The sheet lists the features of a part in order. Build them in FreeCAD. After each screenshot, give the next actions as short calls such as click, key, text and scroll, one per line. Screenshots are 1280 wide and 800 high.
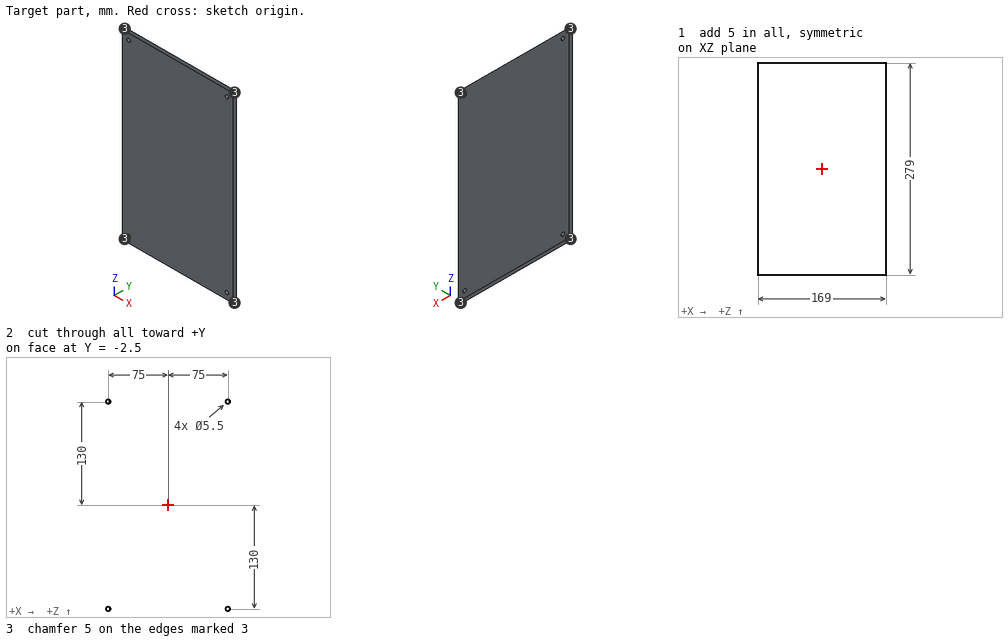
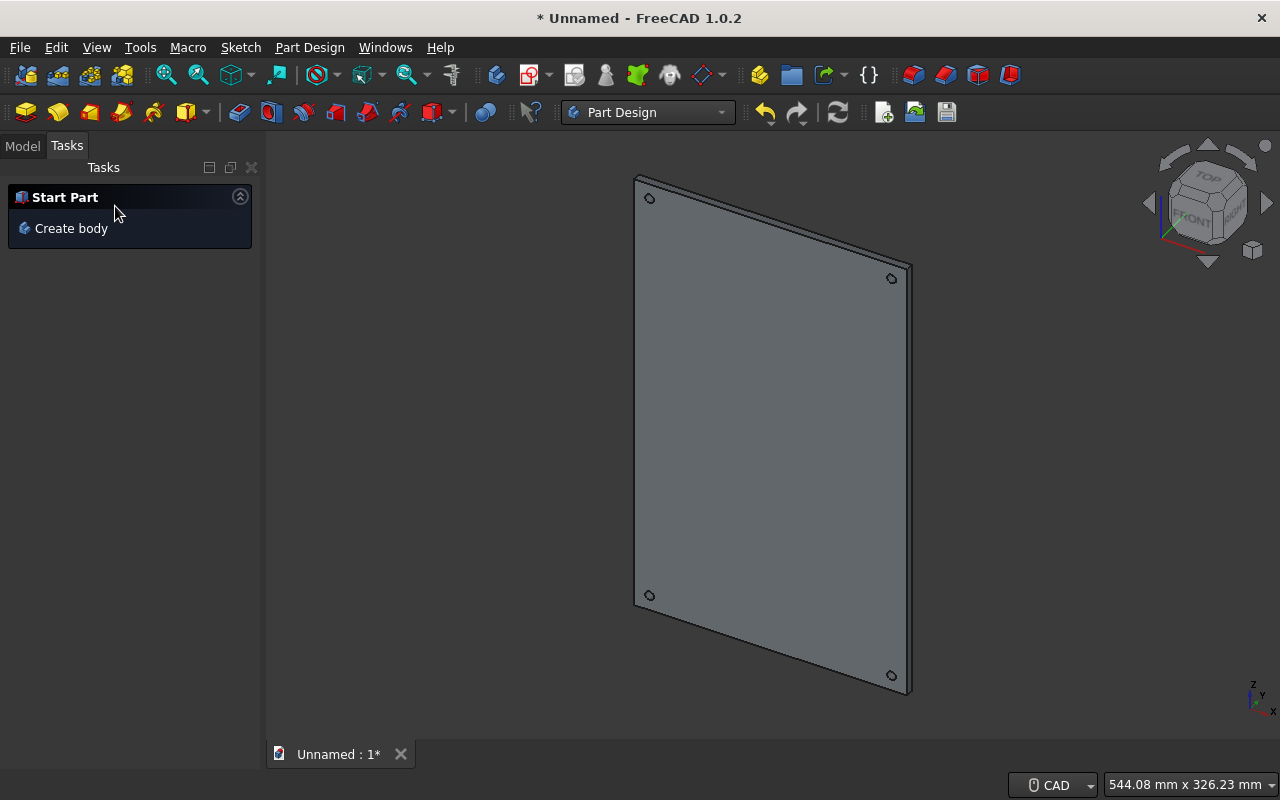
scroll(637, 602, up, 8)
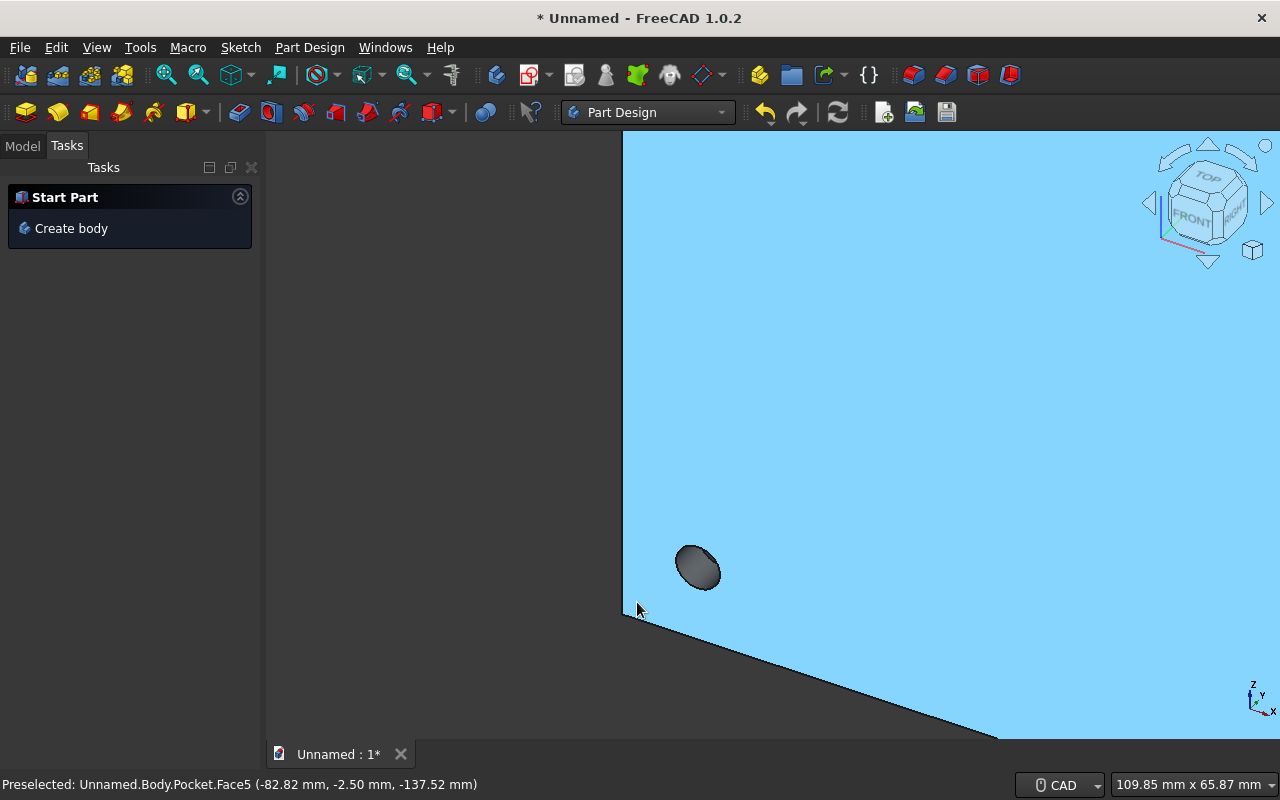
click(168, 76)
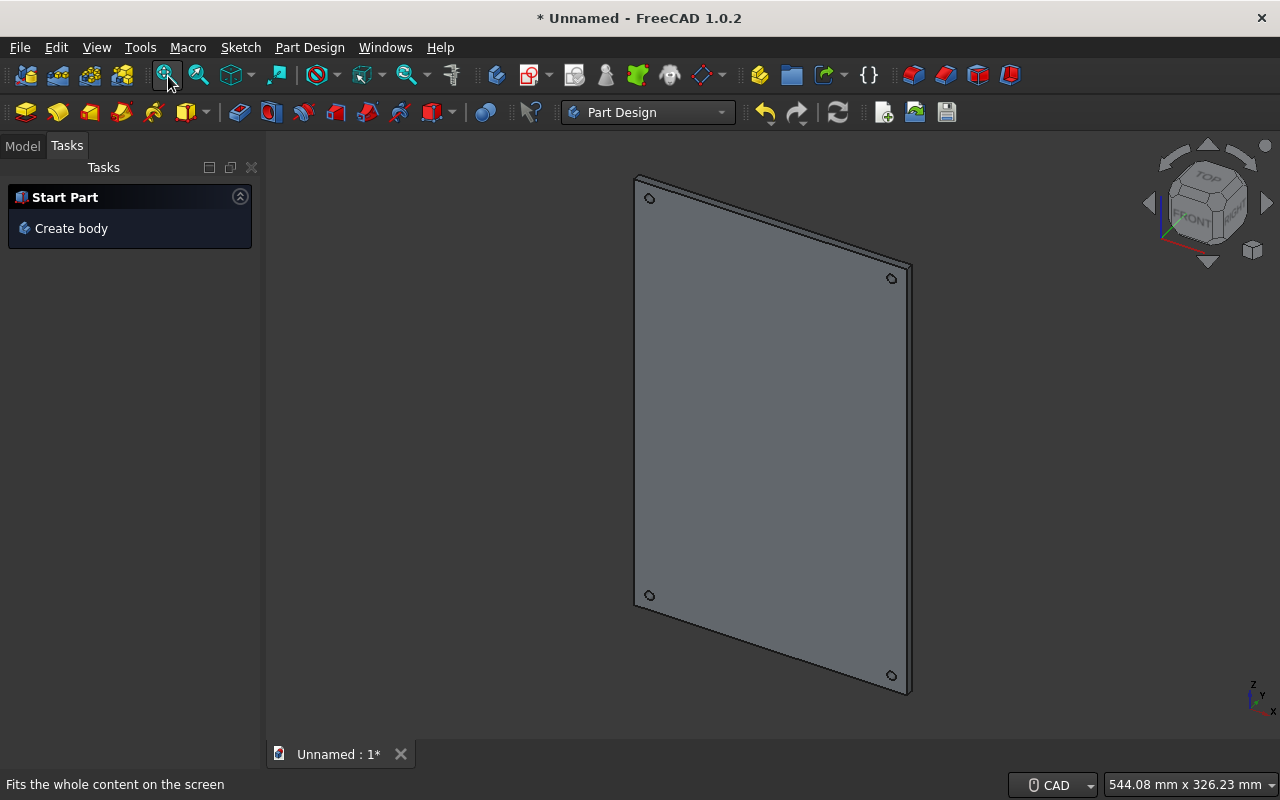
key(0)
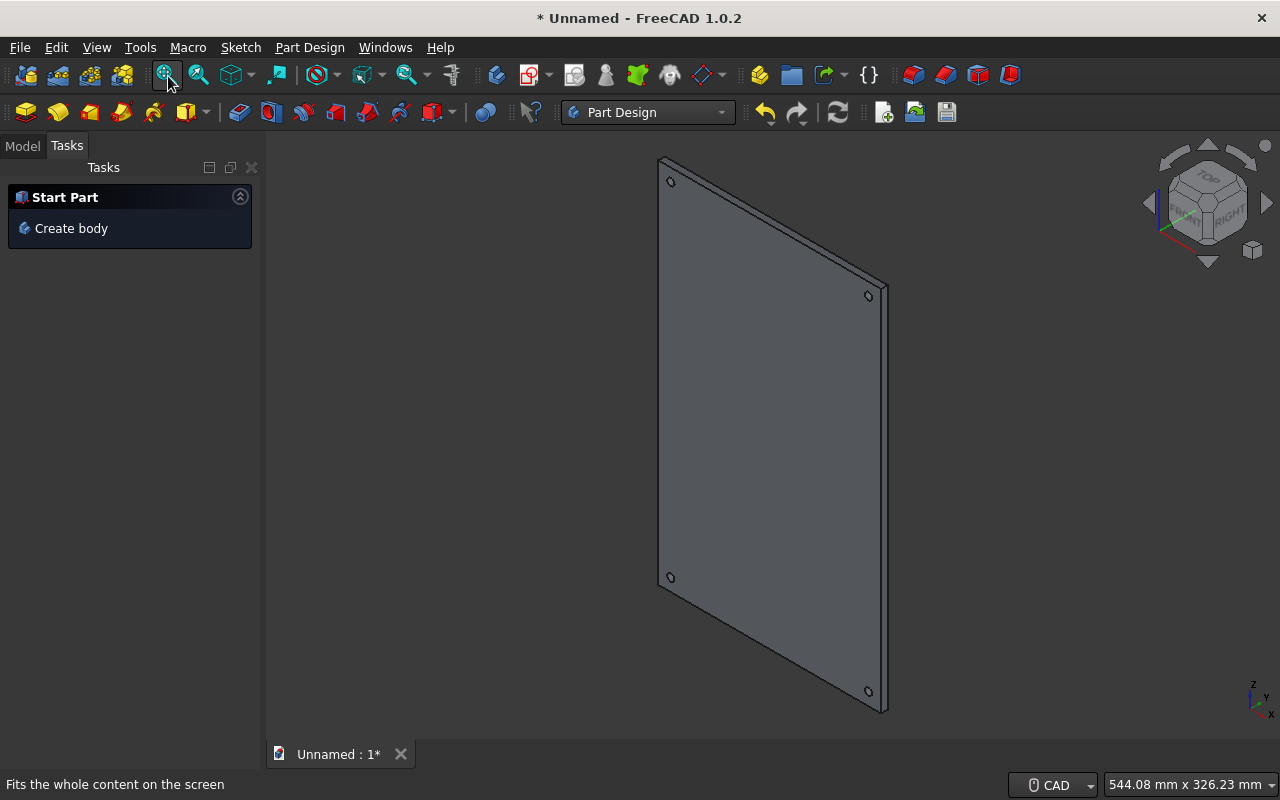
scroll(662, 582, up, 8)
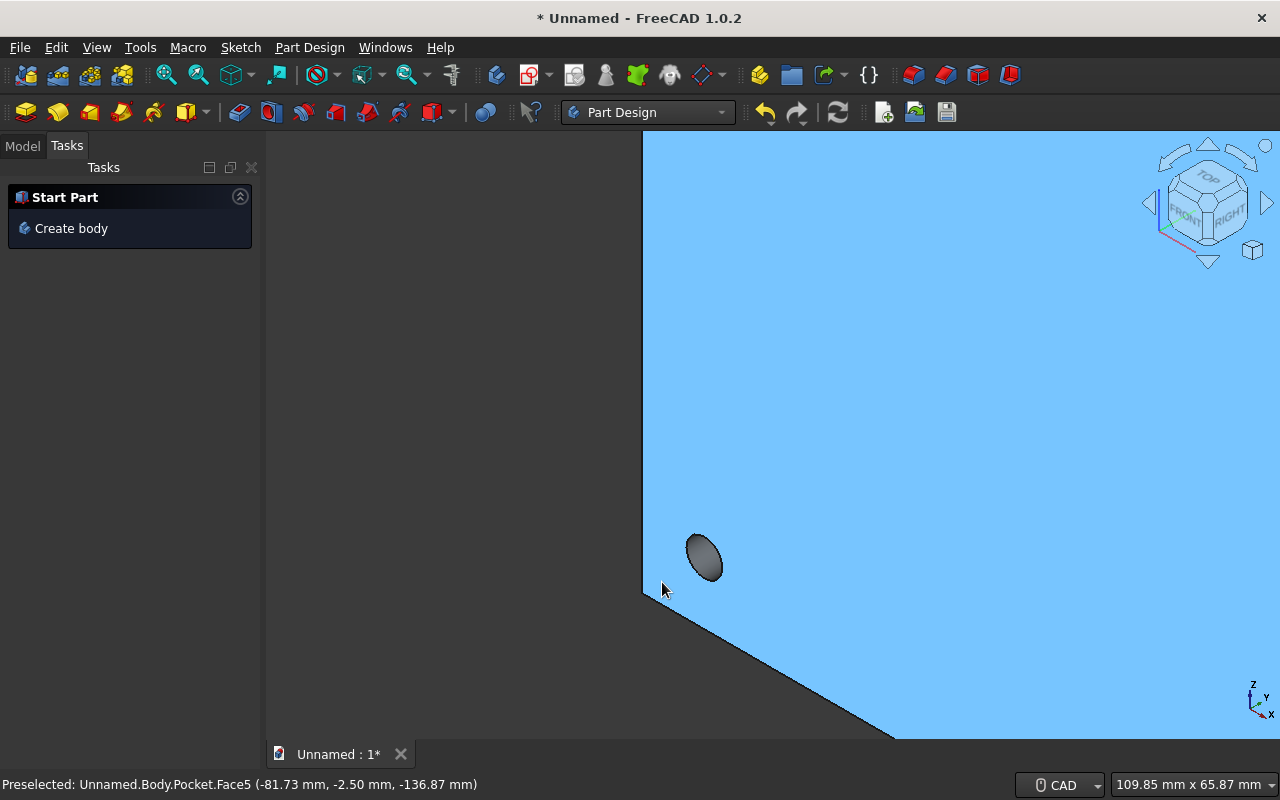
click(168, 76)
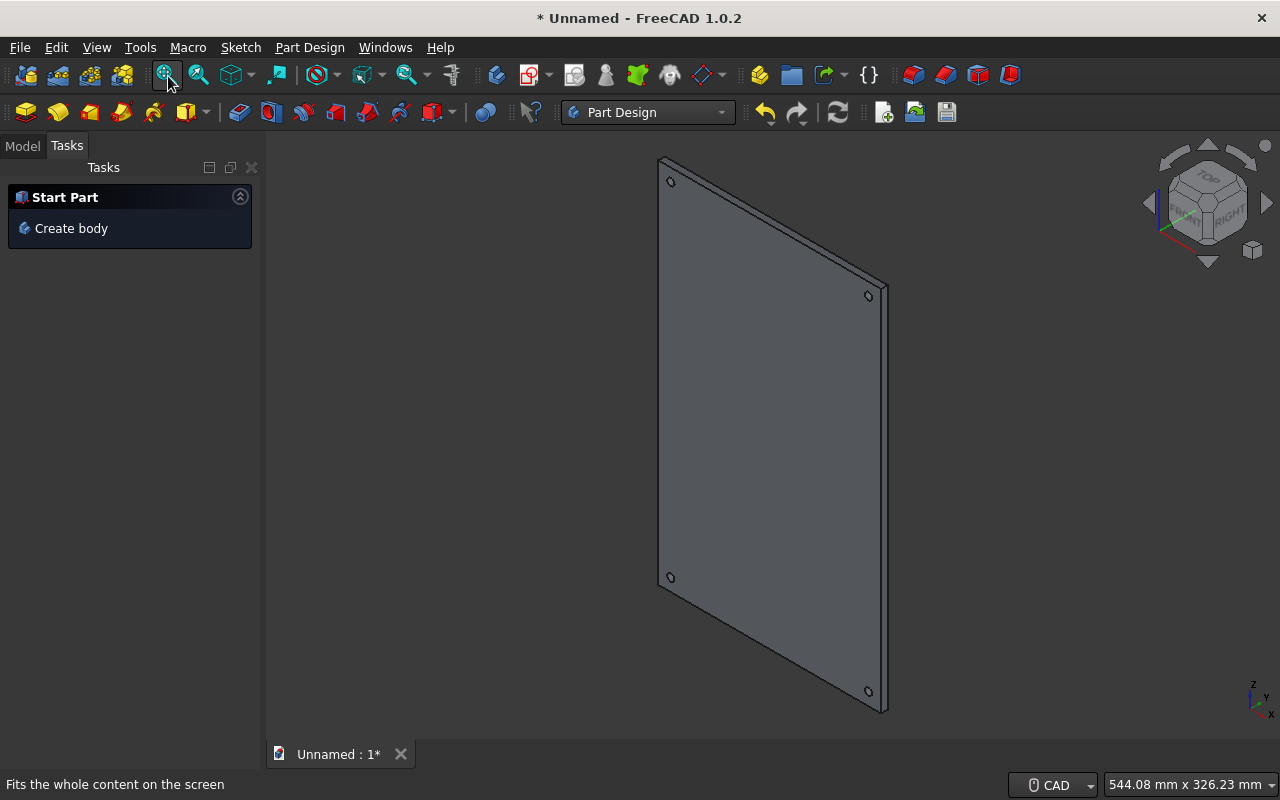
key(2)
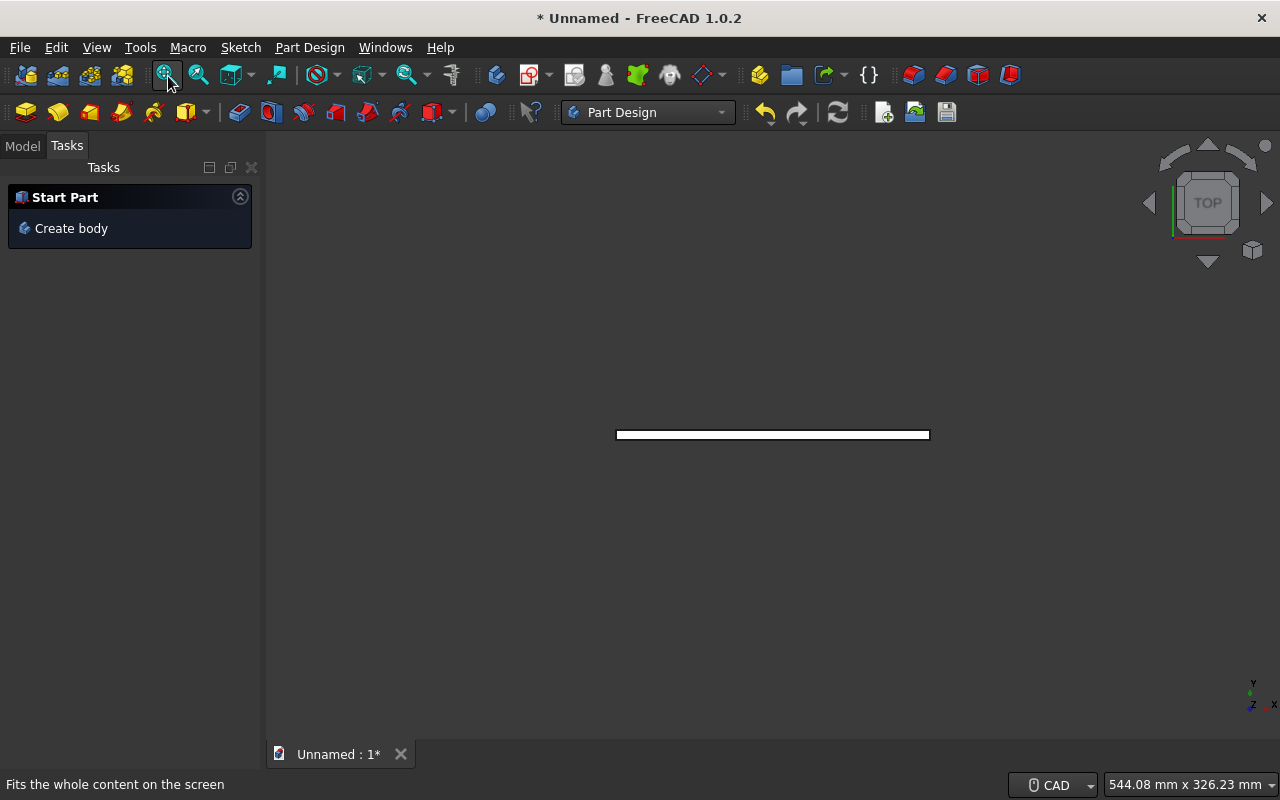
click(168, 76)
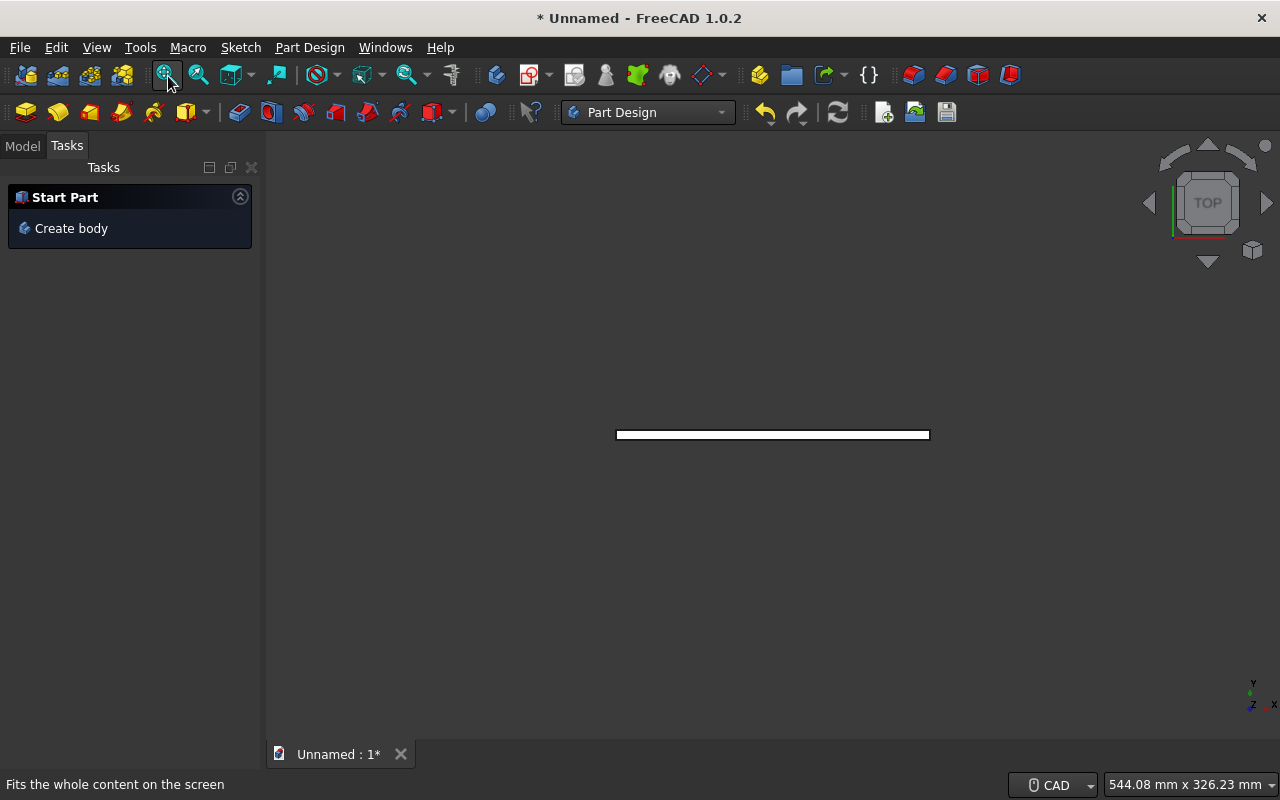
click(930, 436)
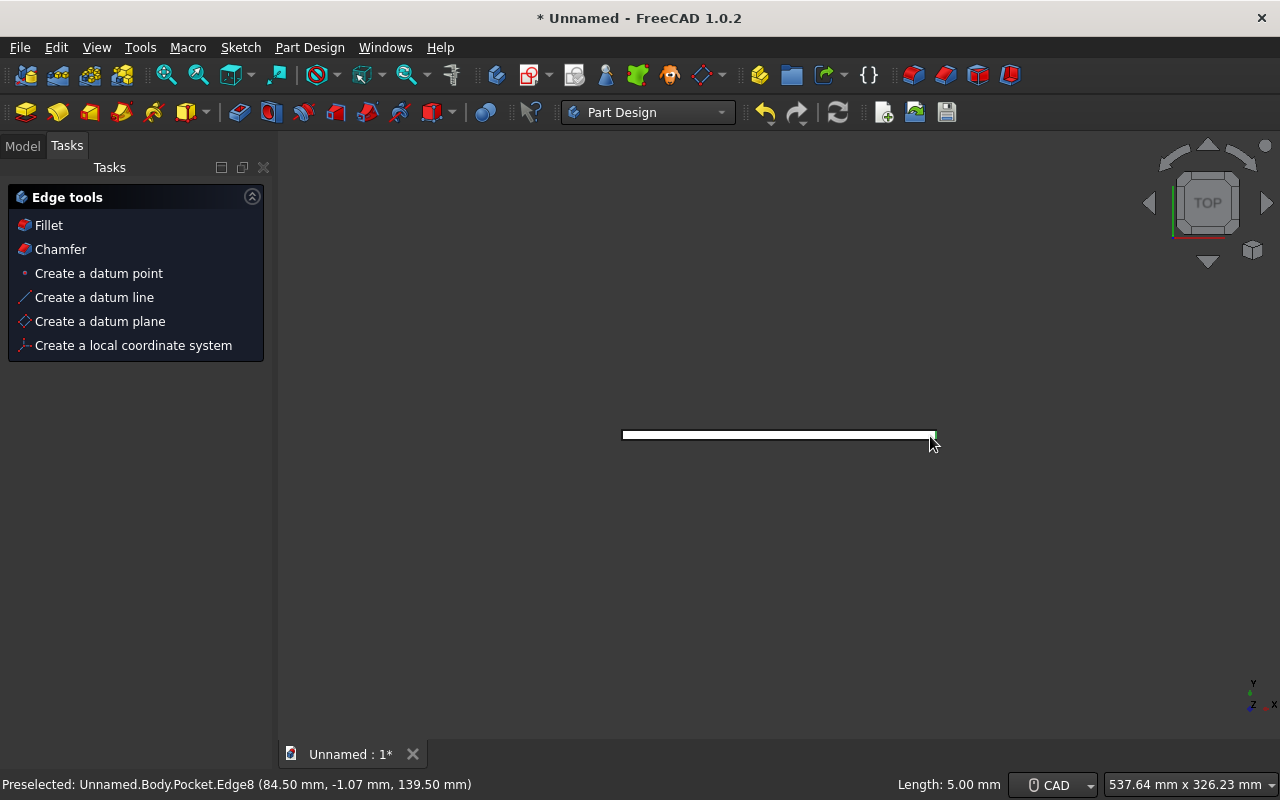
click(622, 436, ctrl)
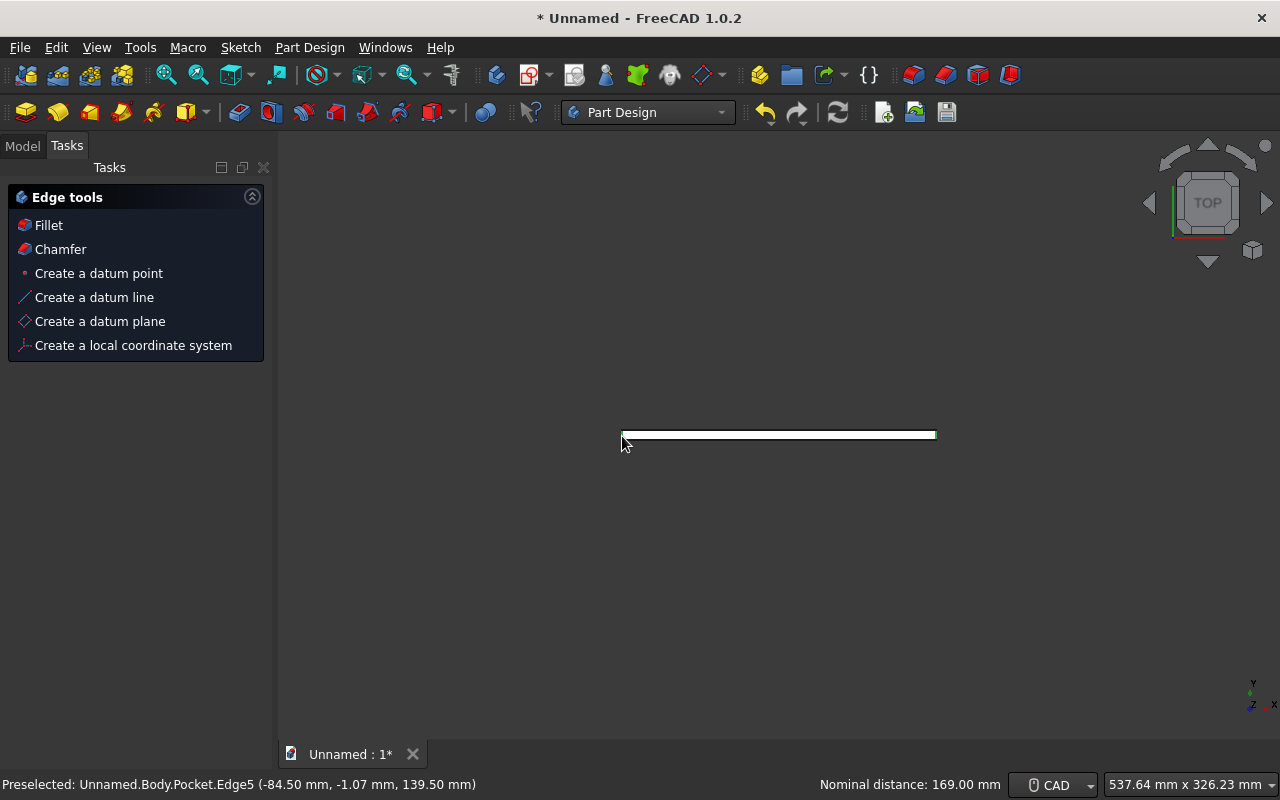
scroll(622, 434, up, 8)